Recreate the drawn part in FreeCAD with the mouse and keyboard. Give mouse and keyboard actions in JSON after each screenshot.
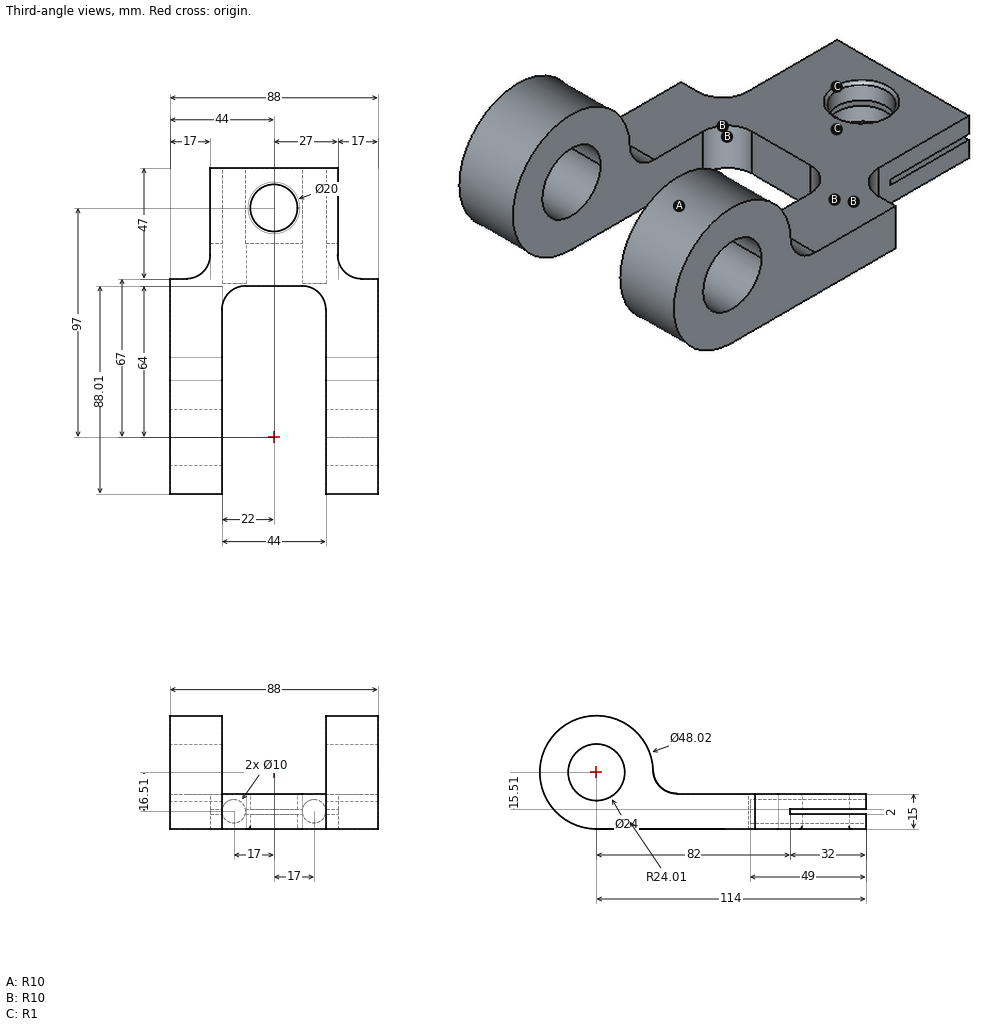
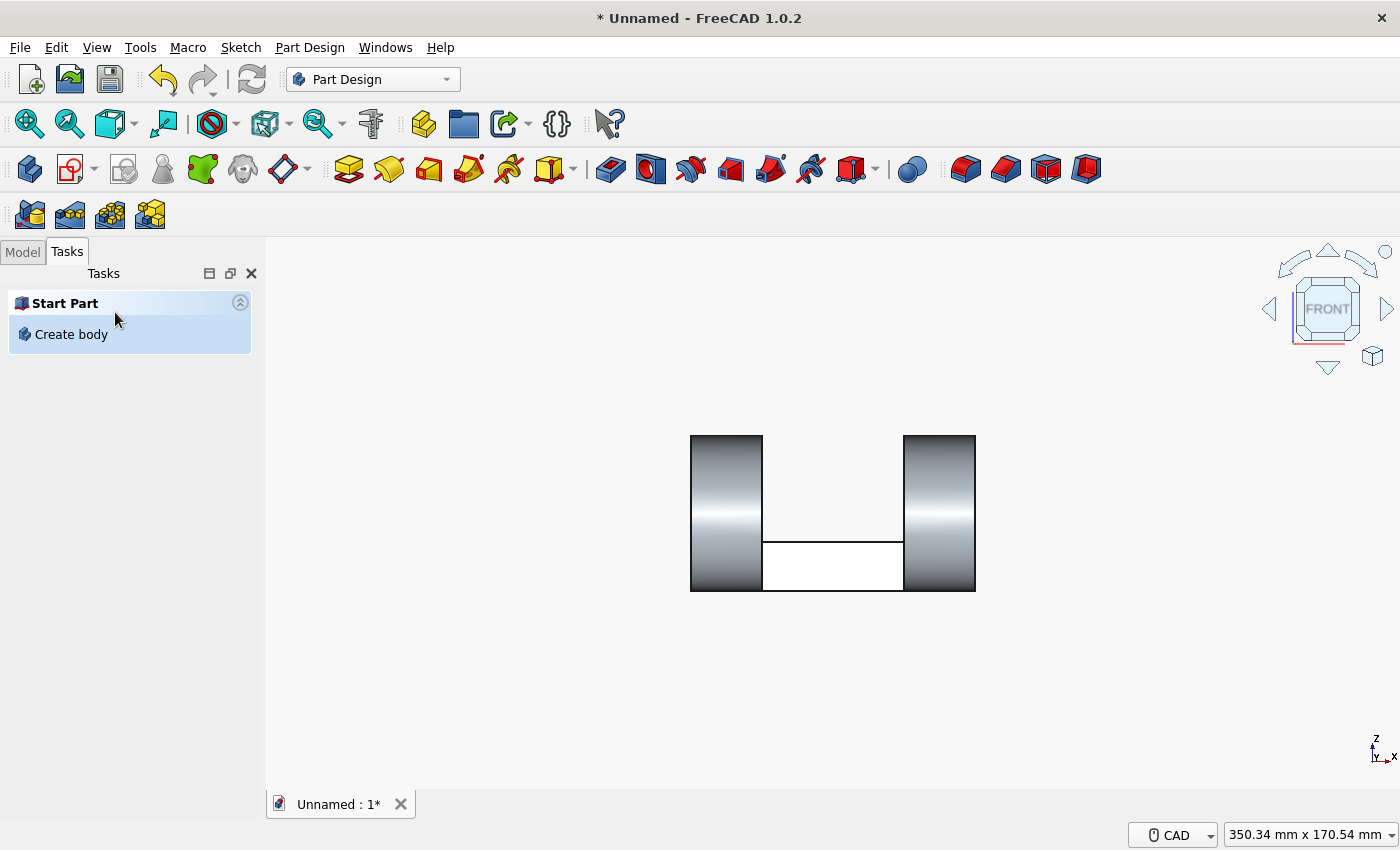
{"action": "left_click", "coordinate": [30, 124]}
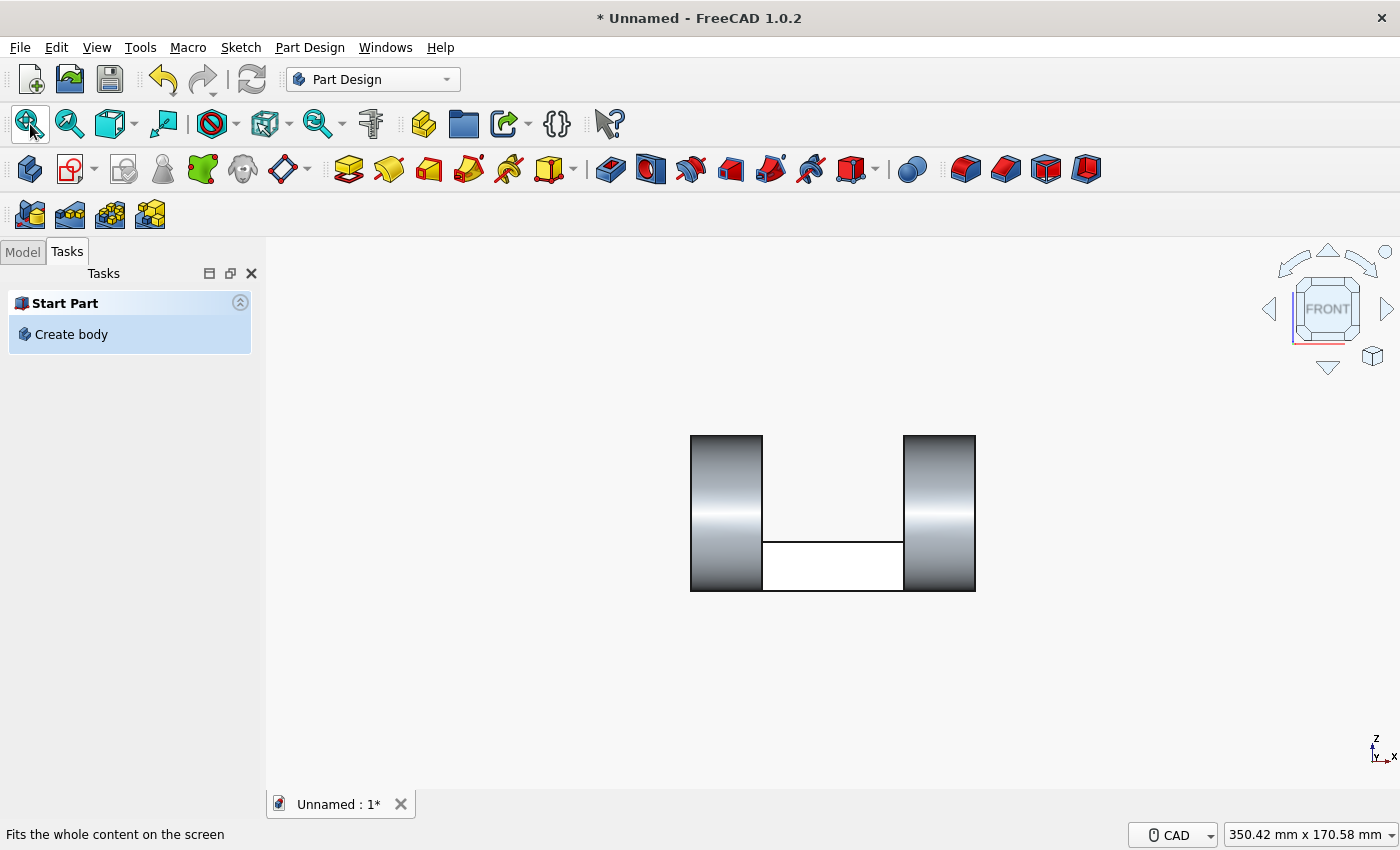
{"action": "key", "text": "3"}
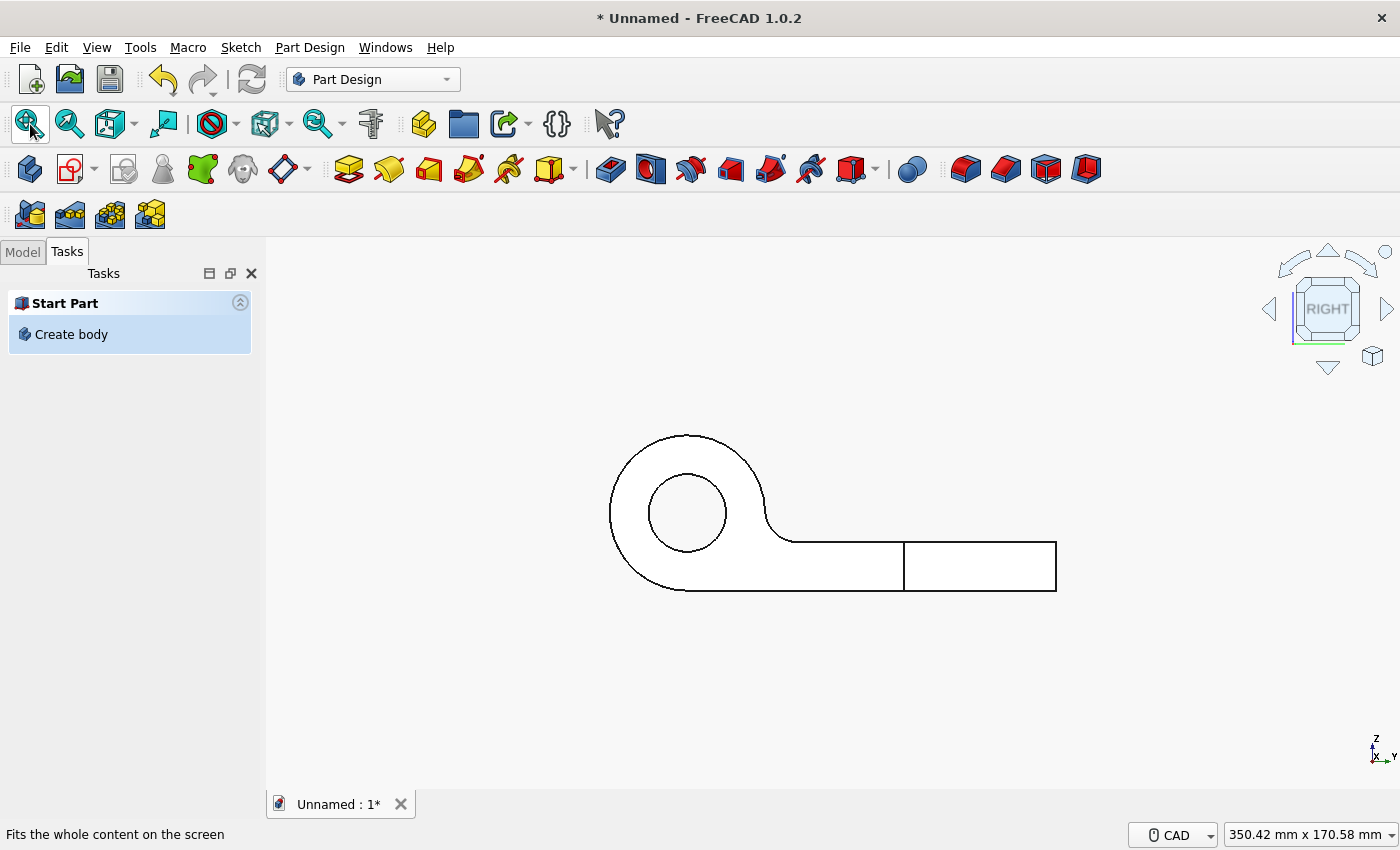
{"action": "left_click", "coordinate": [30, 124]}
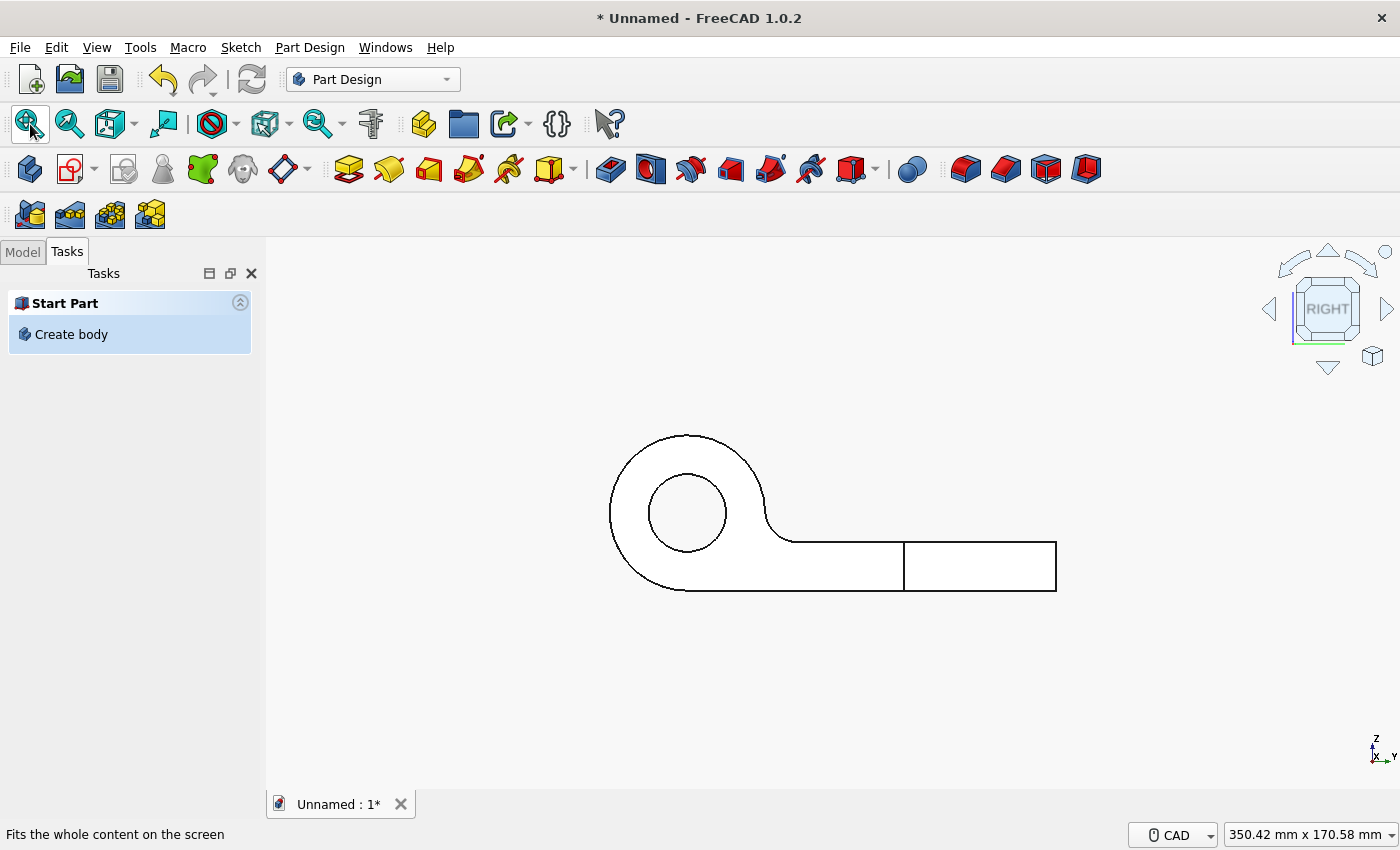
{"action": "key", "text": "5"}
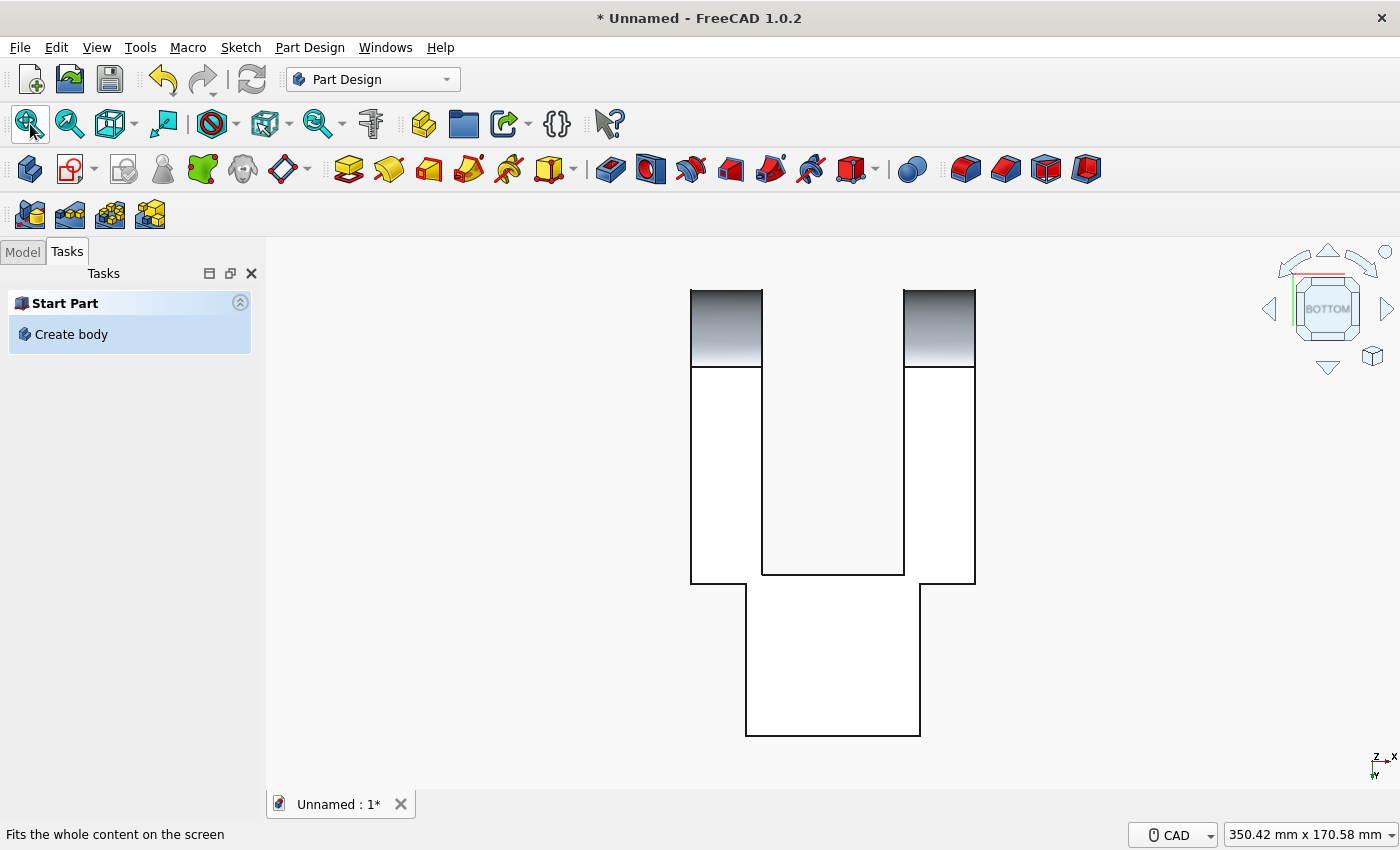
{"action": "key", "text": "4"}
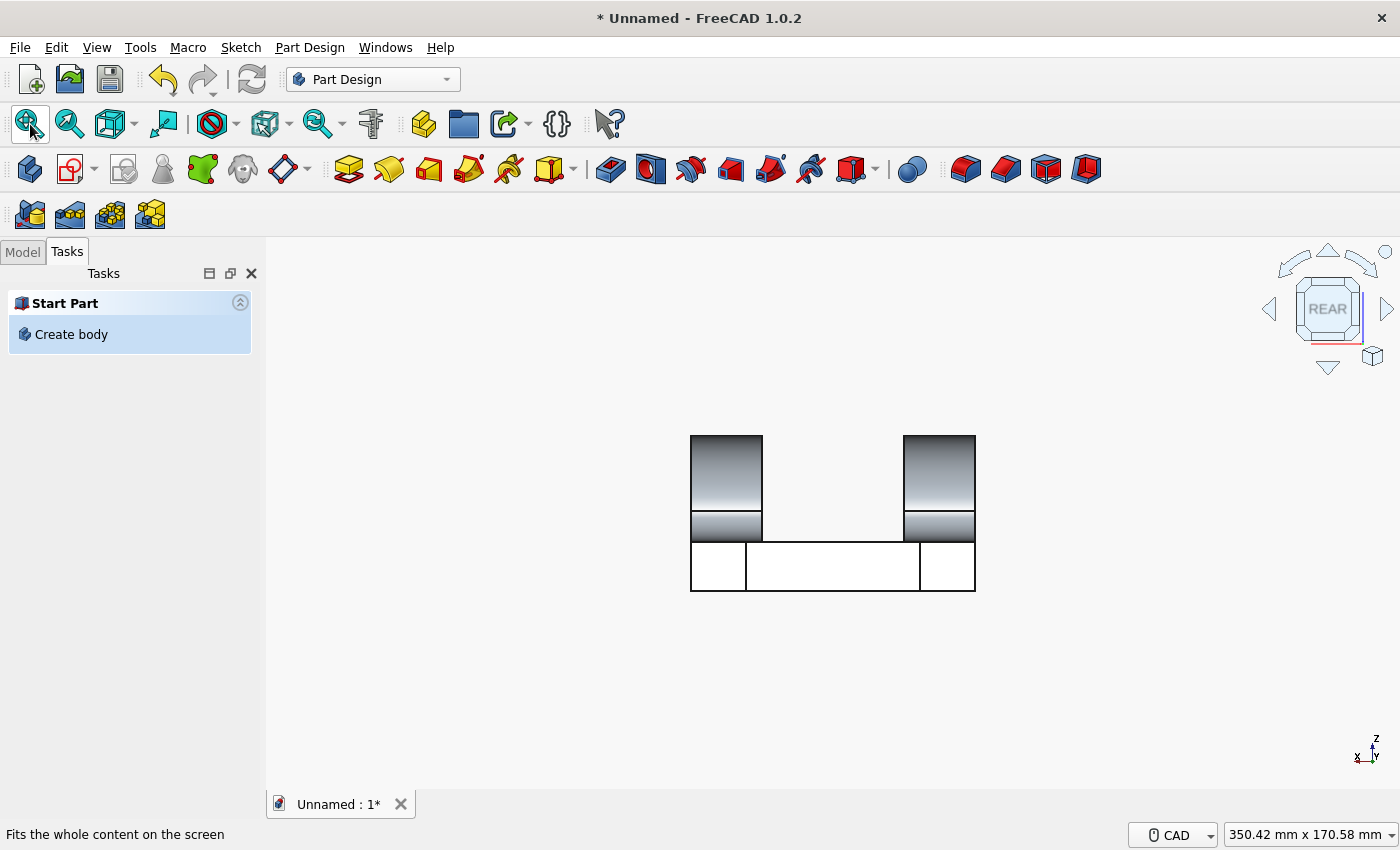
{"action": "left_click", "coordinate": [30, 124]}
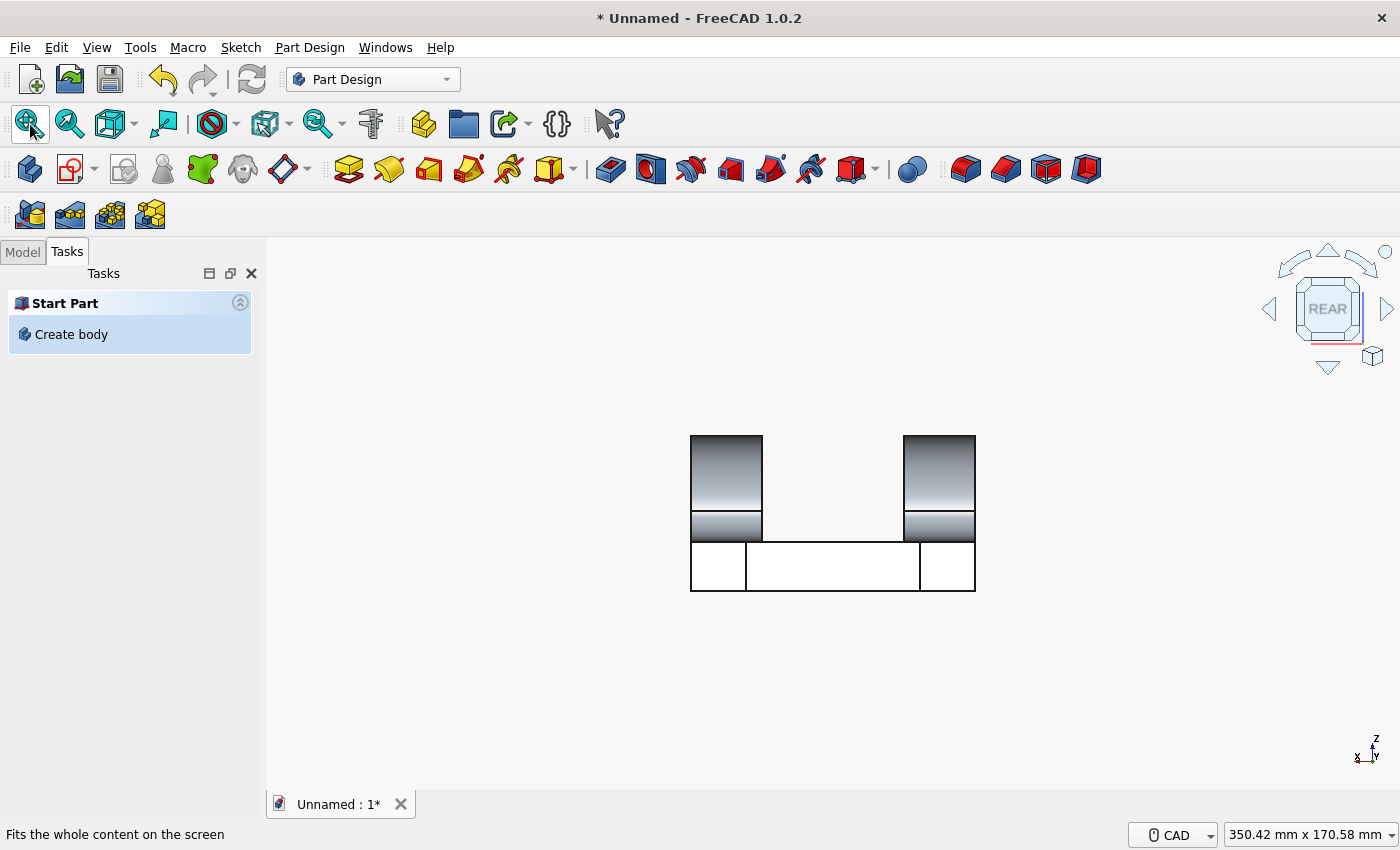
{"action": "key", "text": "6"}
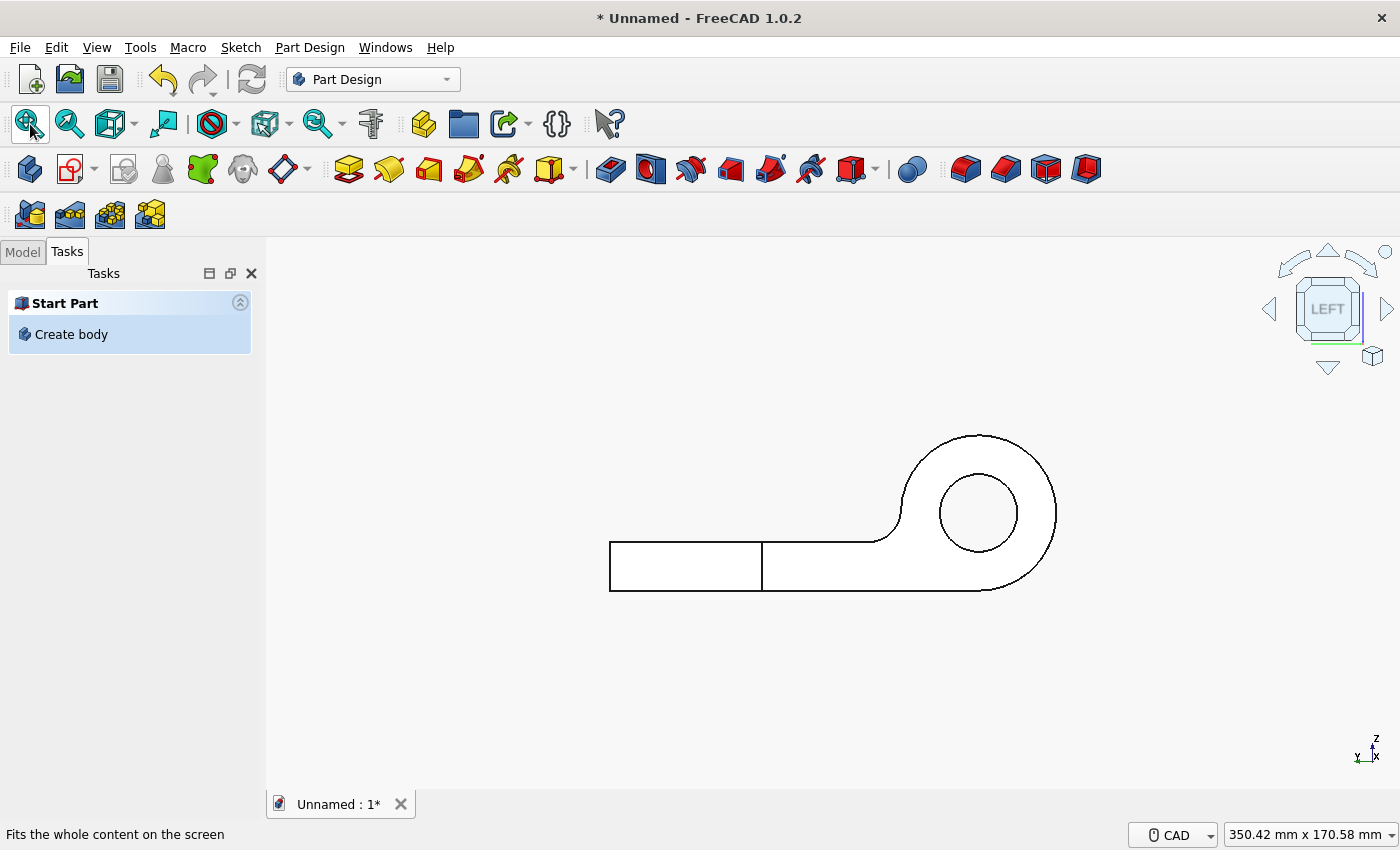
{"action": "left_click", "coordinate": [30, 124]}